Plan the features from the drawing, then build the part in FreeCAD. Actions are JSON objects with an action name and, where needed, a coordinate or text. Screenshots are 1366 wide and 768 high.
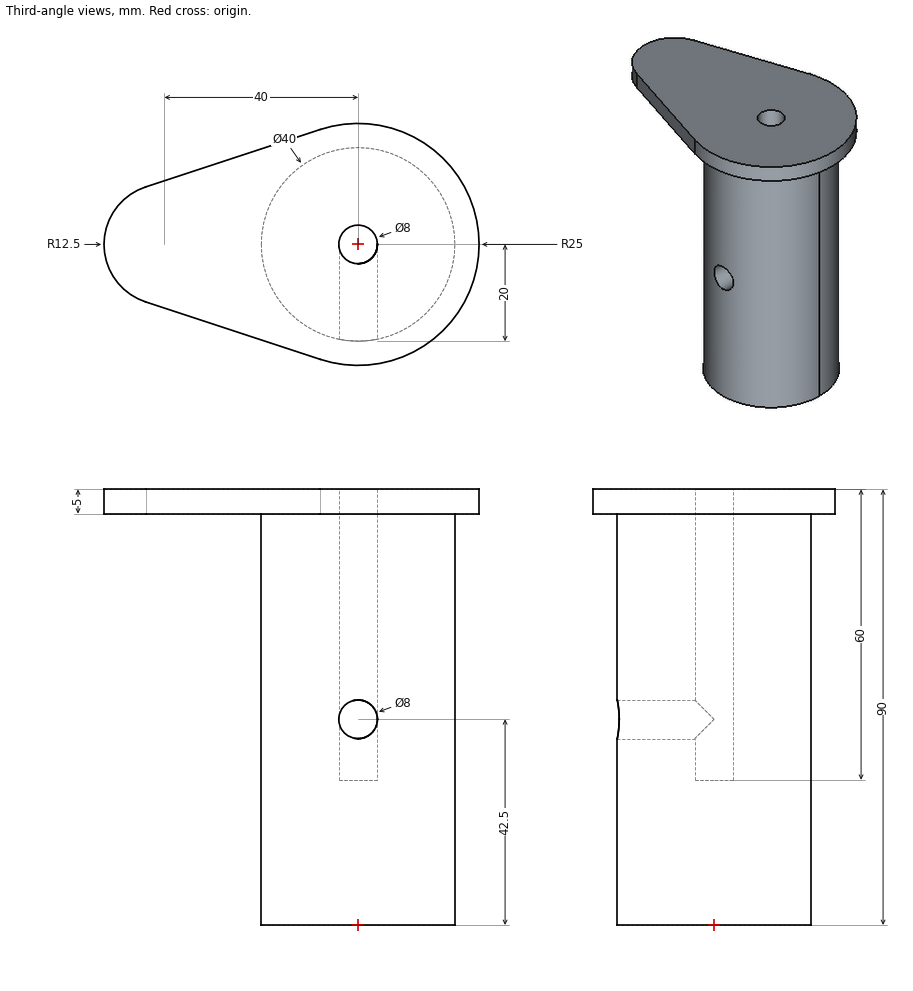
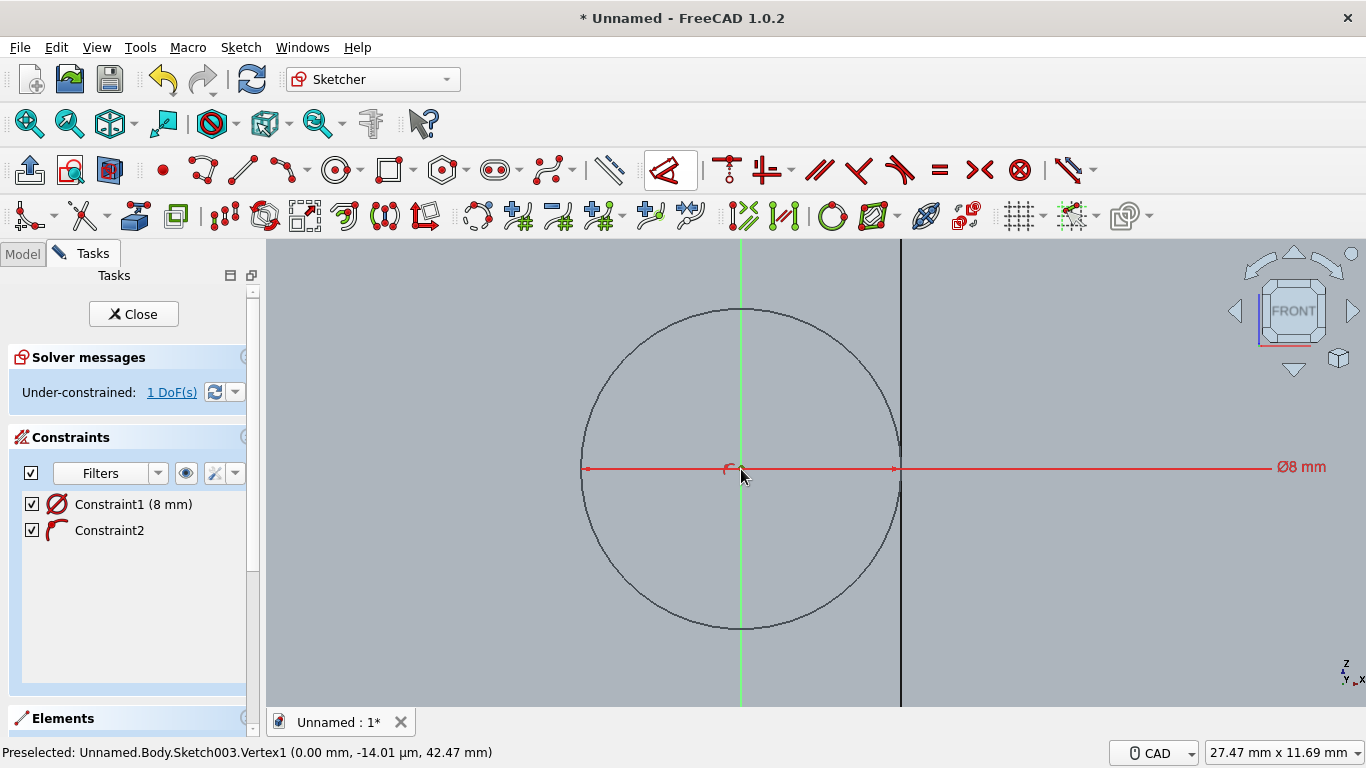
{"action": "key", "text": "i"}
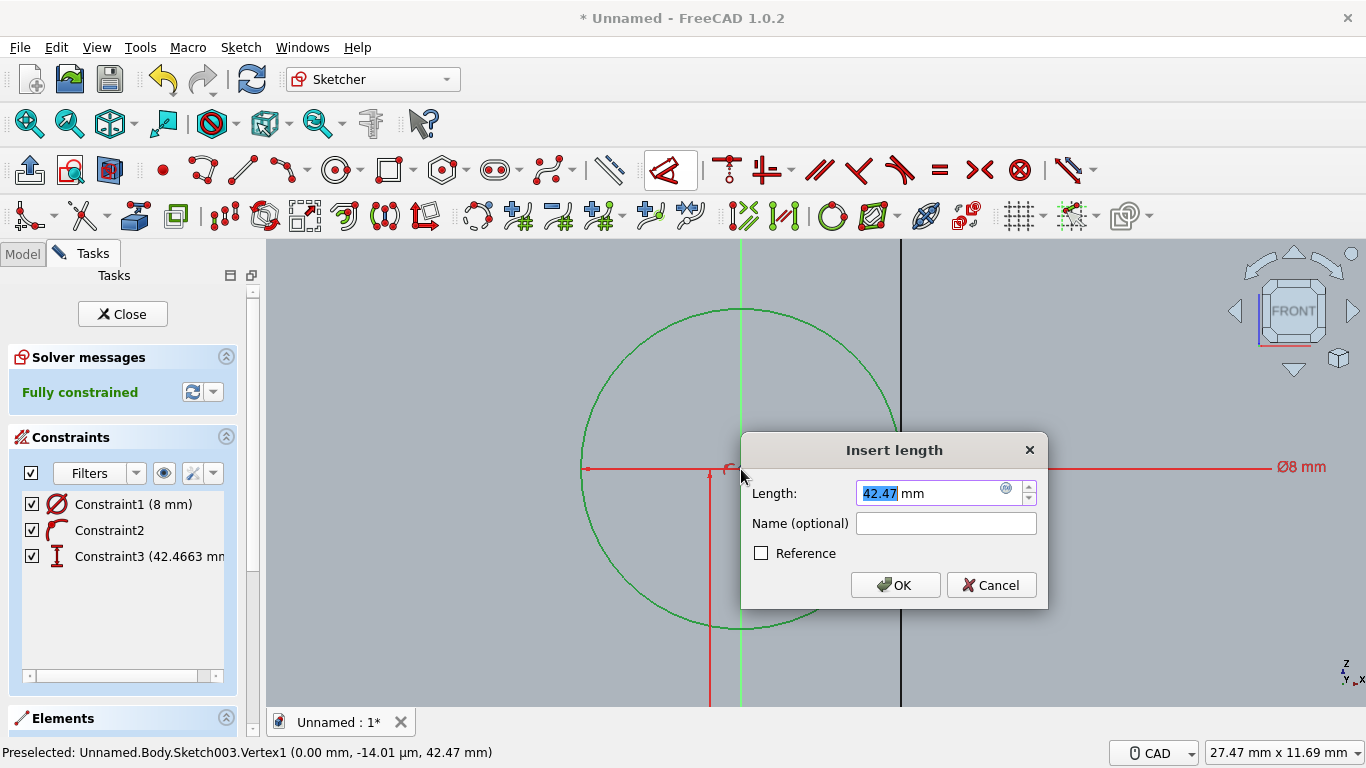
{"action": "type", "text": "42.5"}
{"action": "key", "text": "Return"}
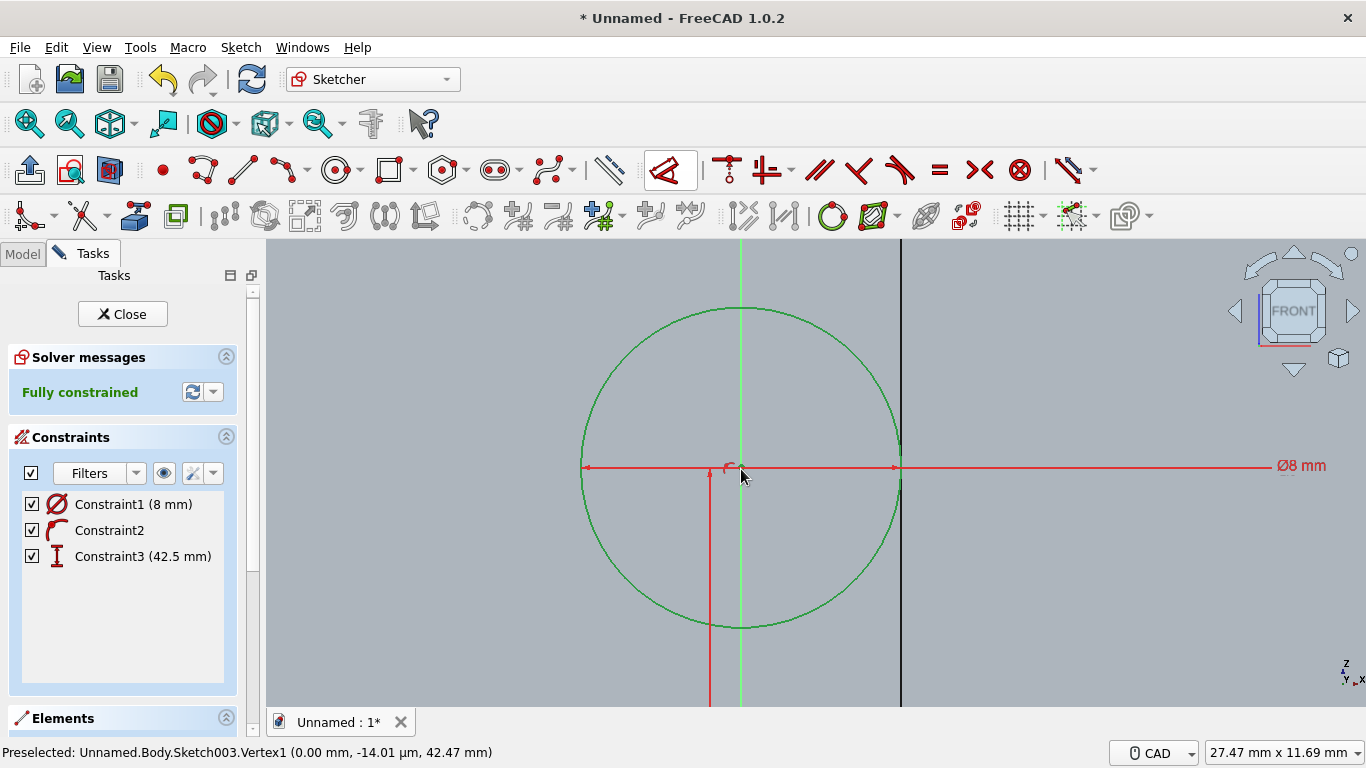
{"action": "left_click", "coordinate": [123, 314]}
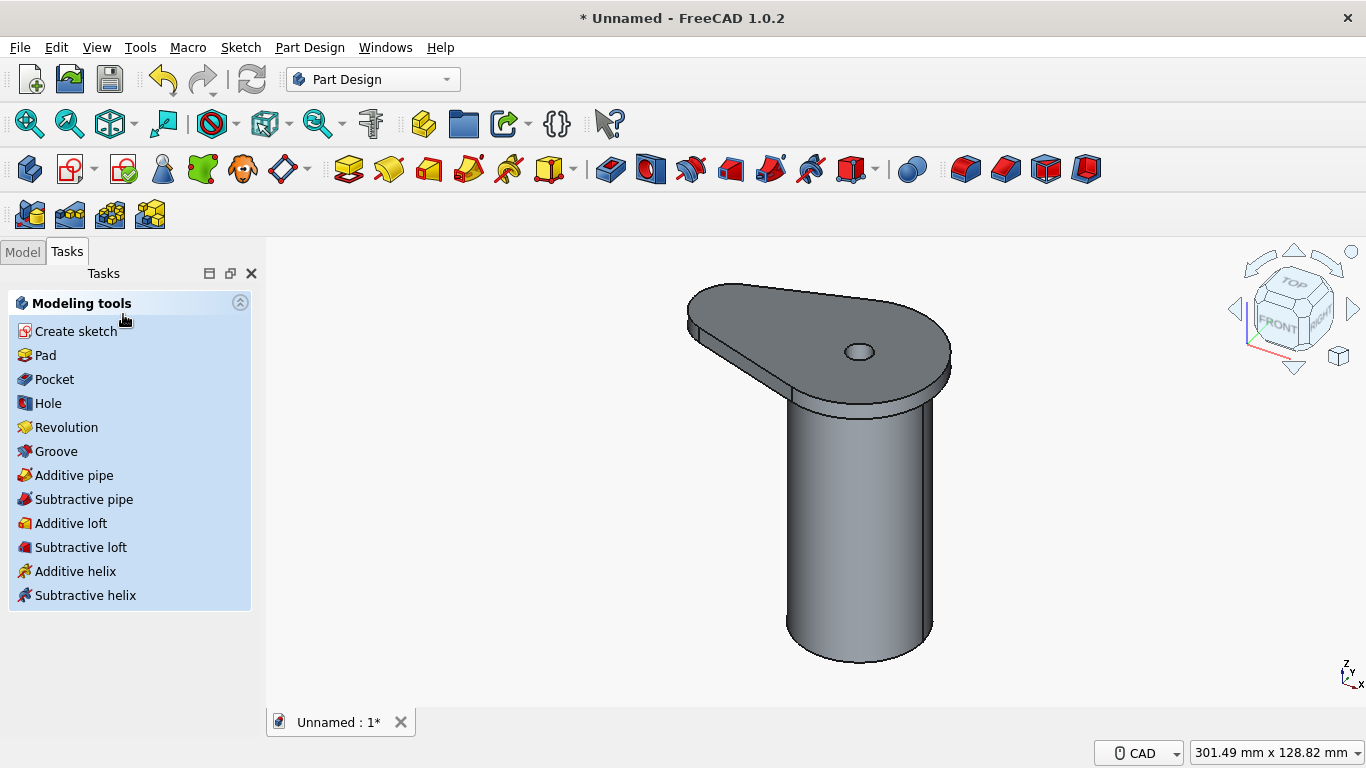
{"action": "left_click", "coordinate": [612, 170]}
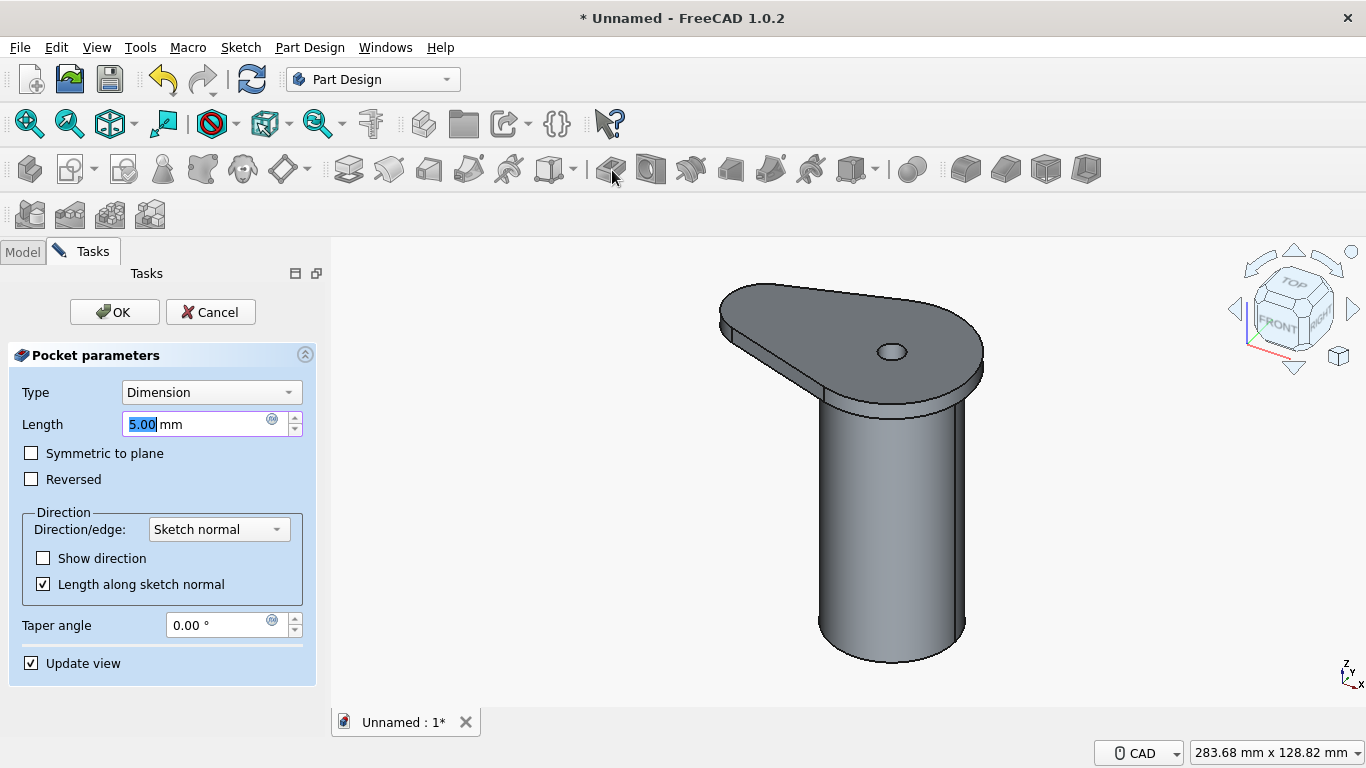
{"action": "type", "text": "20"}
{"action": "key", "text": "Tab"}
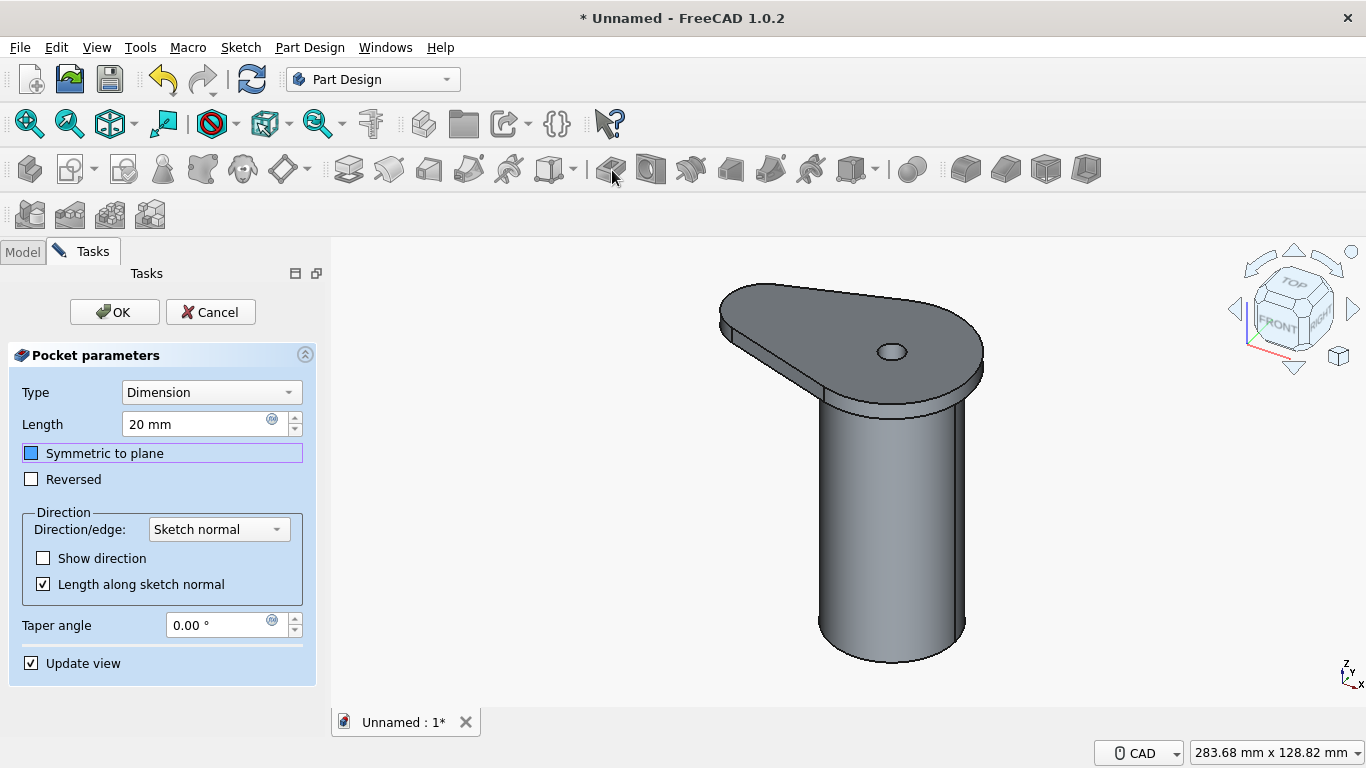
{"action": "left_click", "coordinate": [30, 479]}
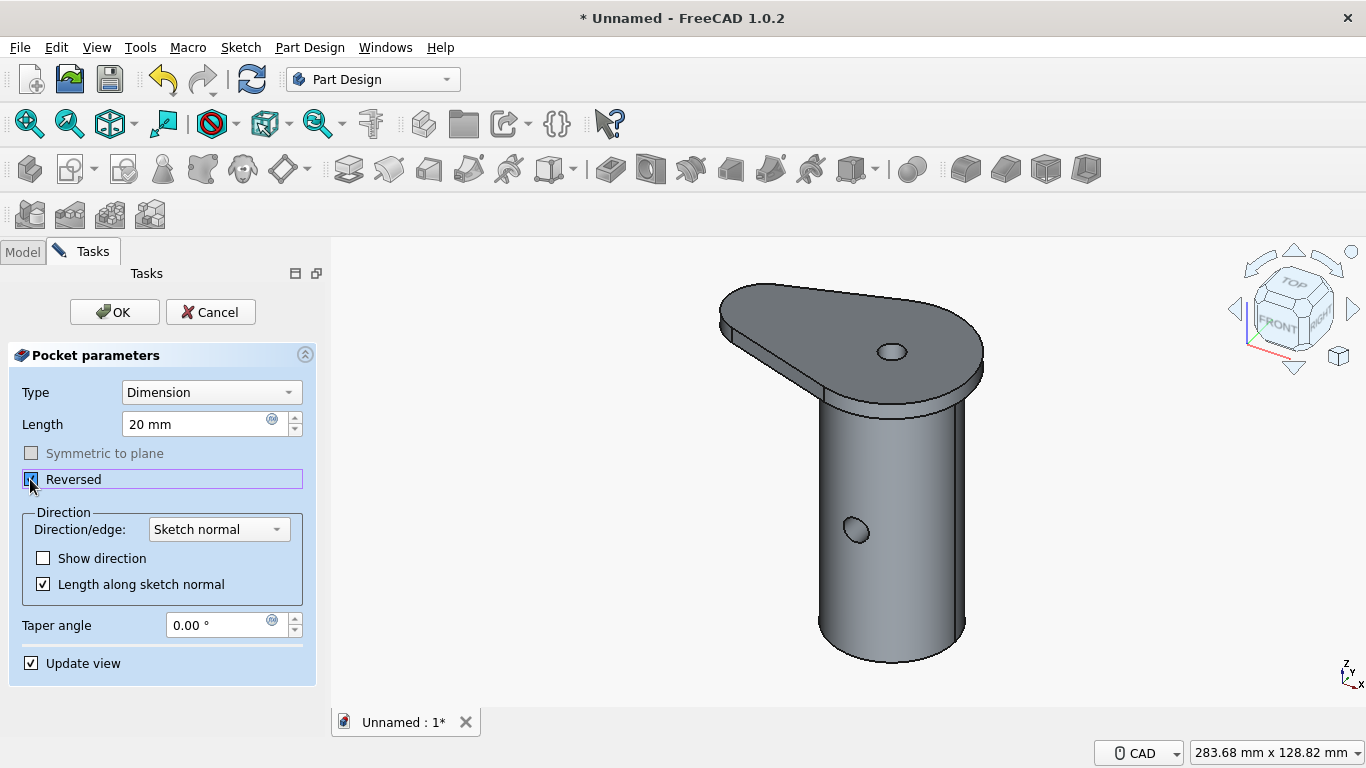
{"action": "left_click", "coordinate": [115, 312]}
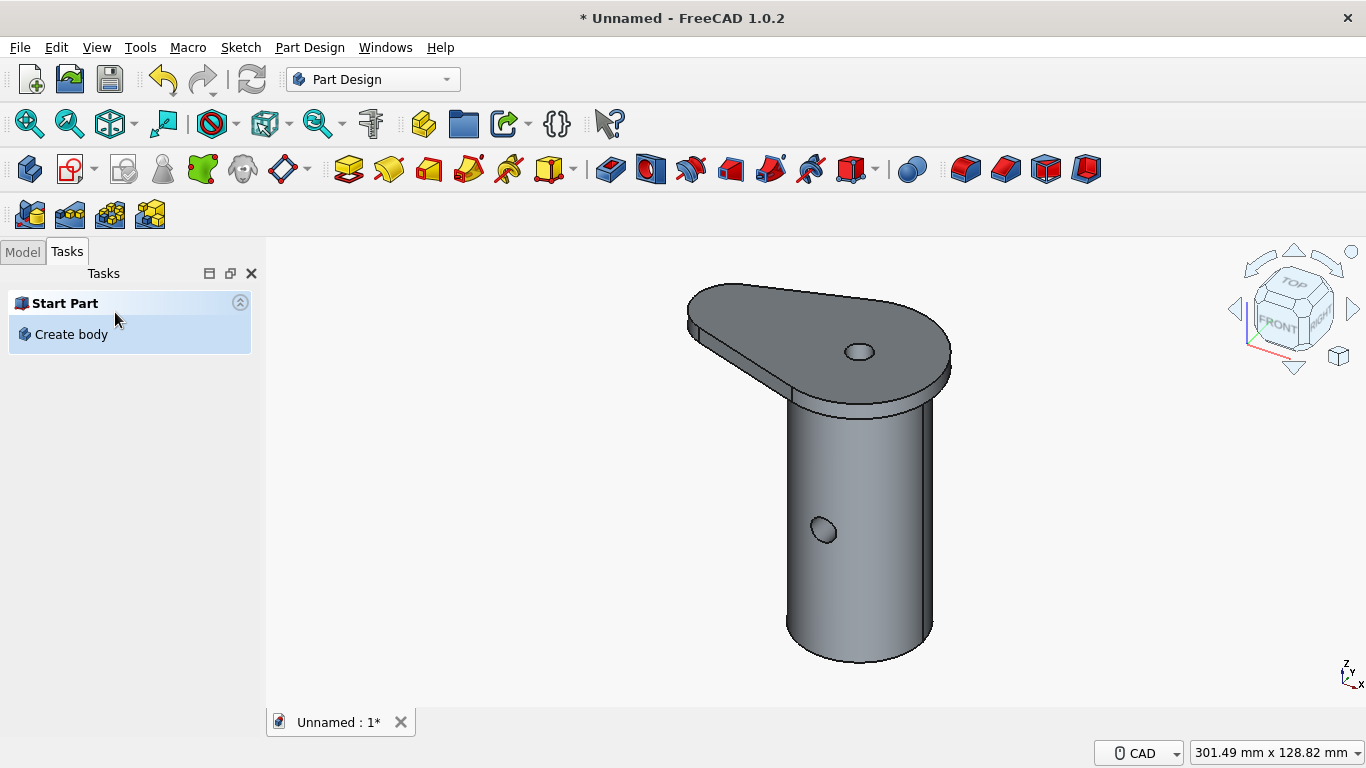
{"action": "key", "text": "0"}